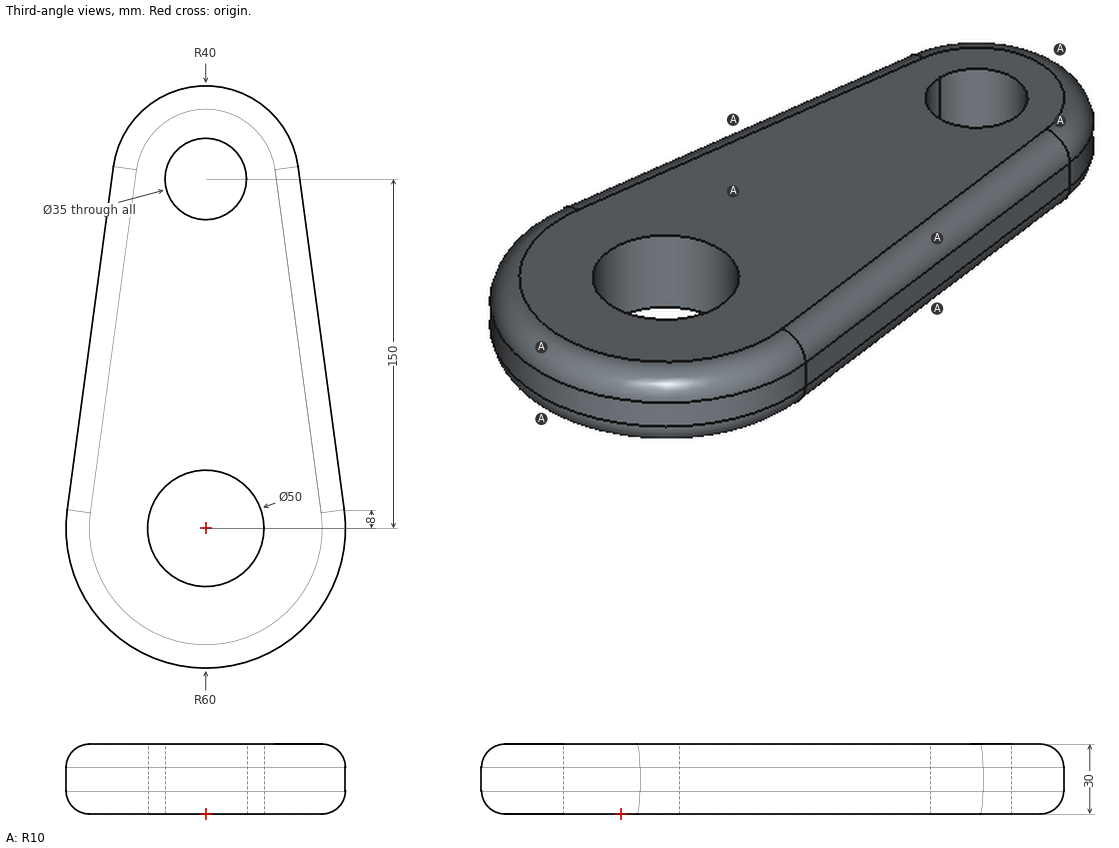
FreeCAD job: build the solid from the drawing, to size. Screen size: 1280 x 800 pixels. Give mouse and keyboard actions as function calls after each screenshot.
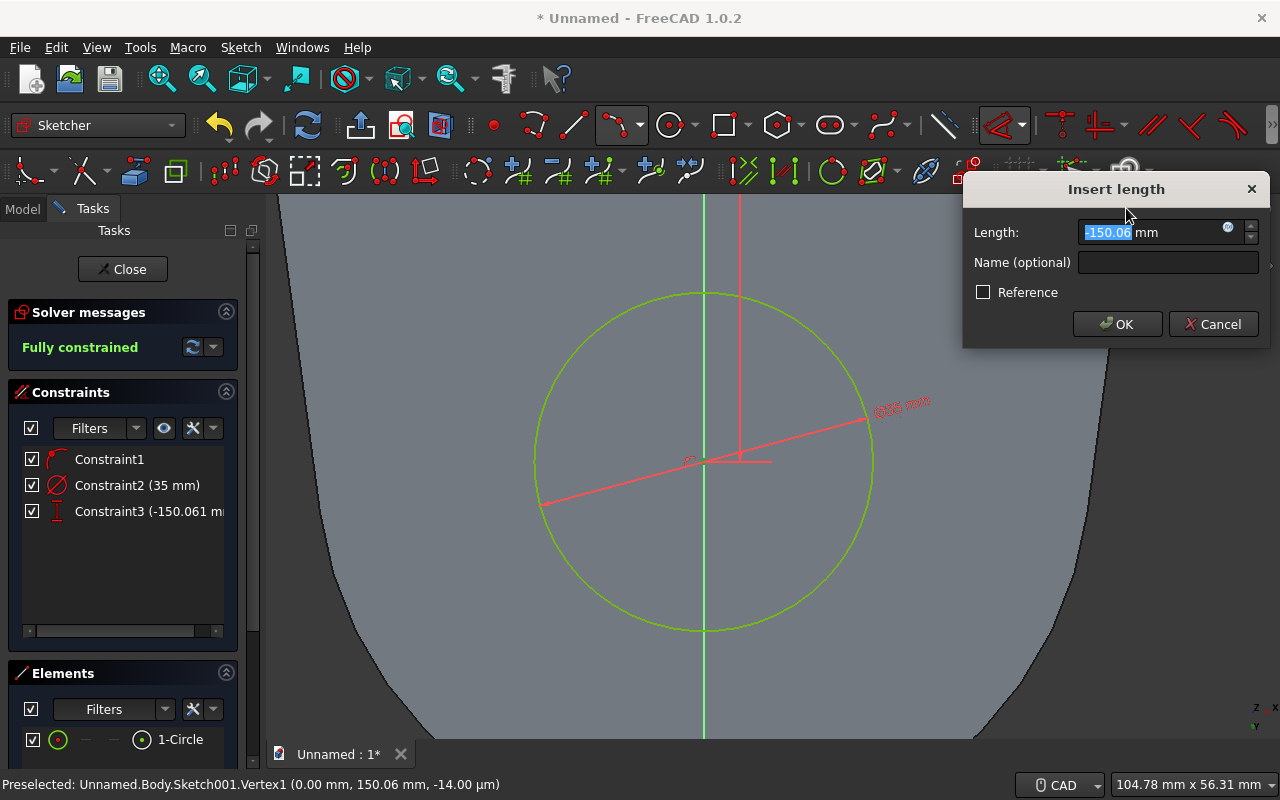
text(-150)
key(Return)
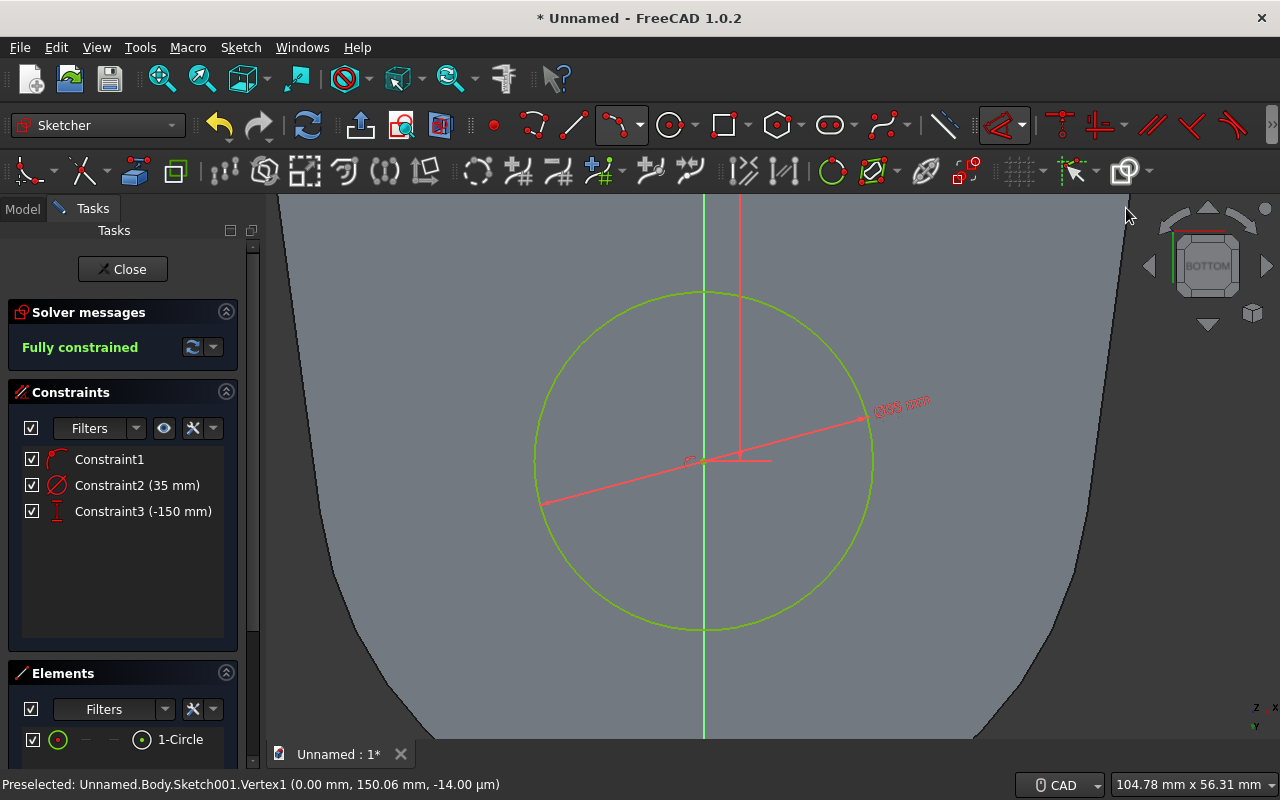
click(123, 269)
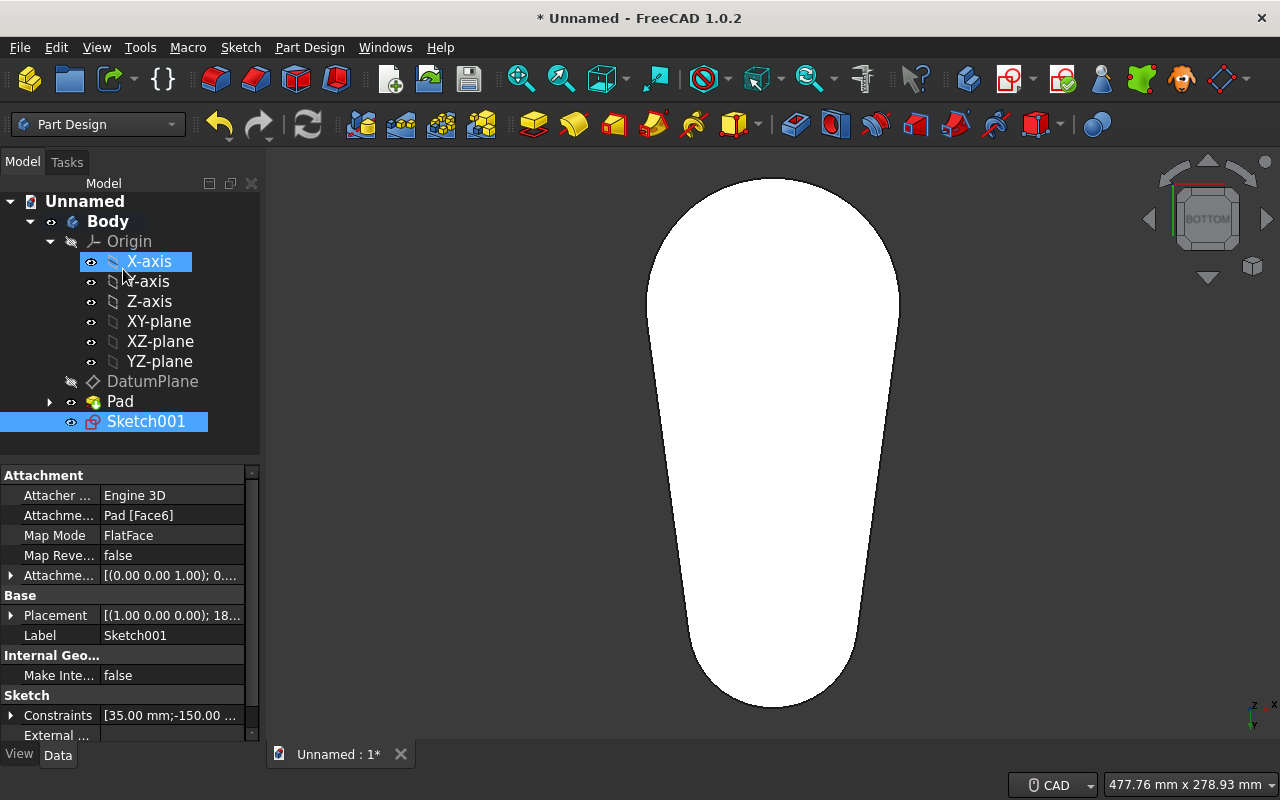
click(836, 124)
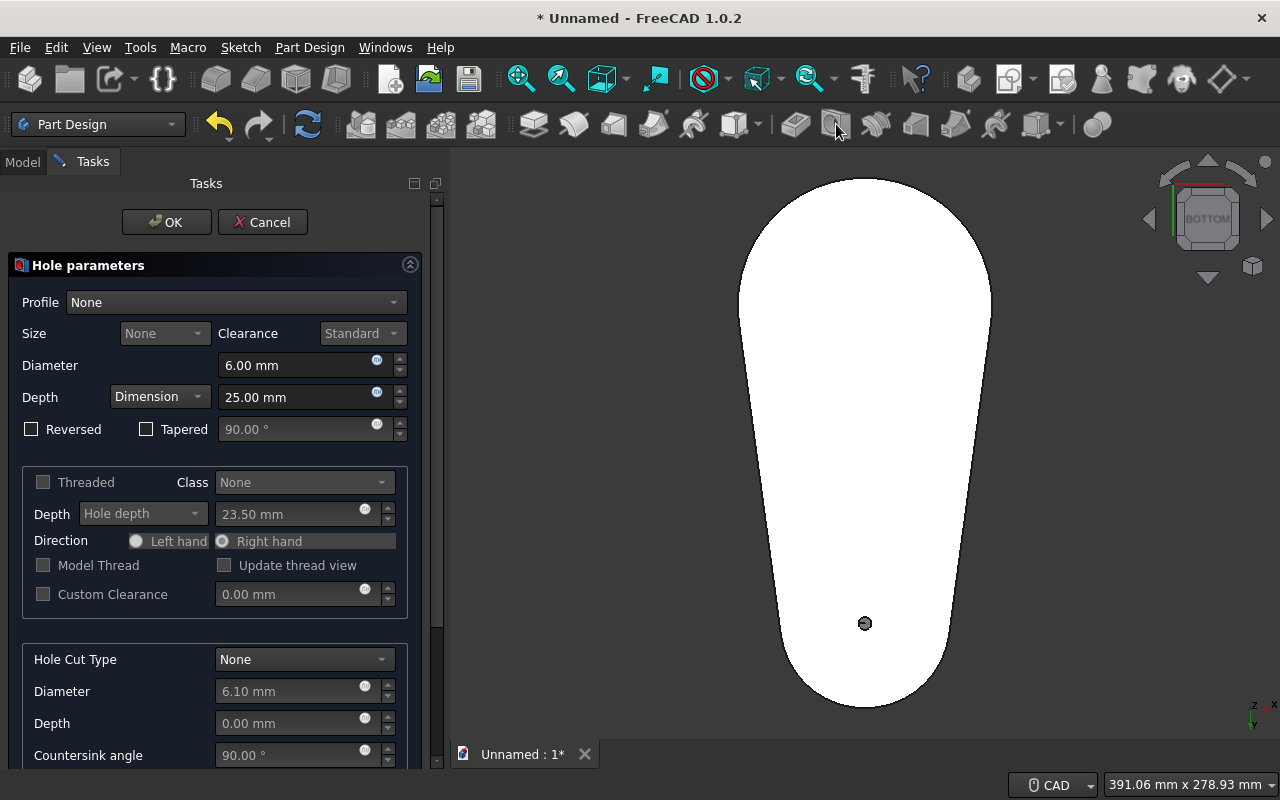
triple_click(305, 365)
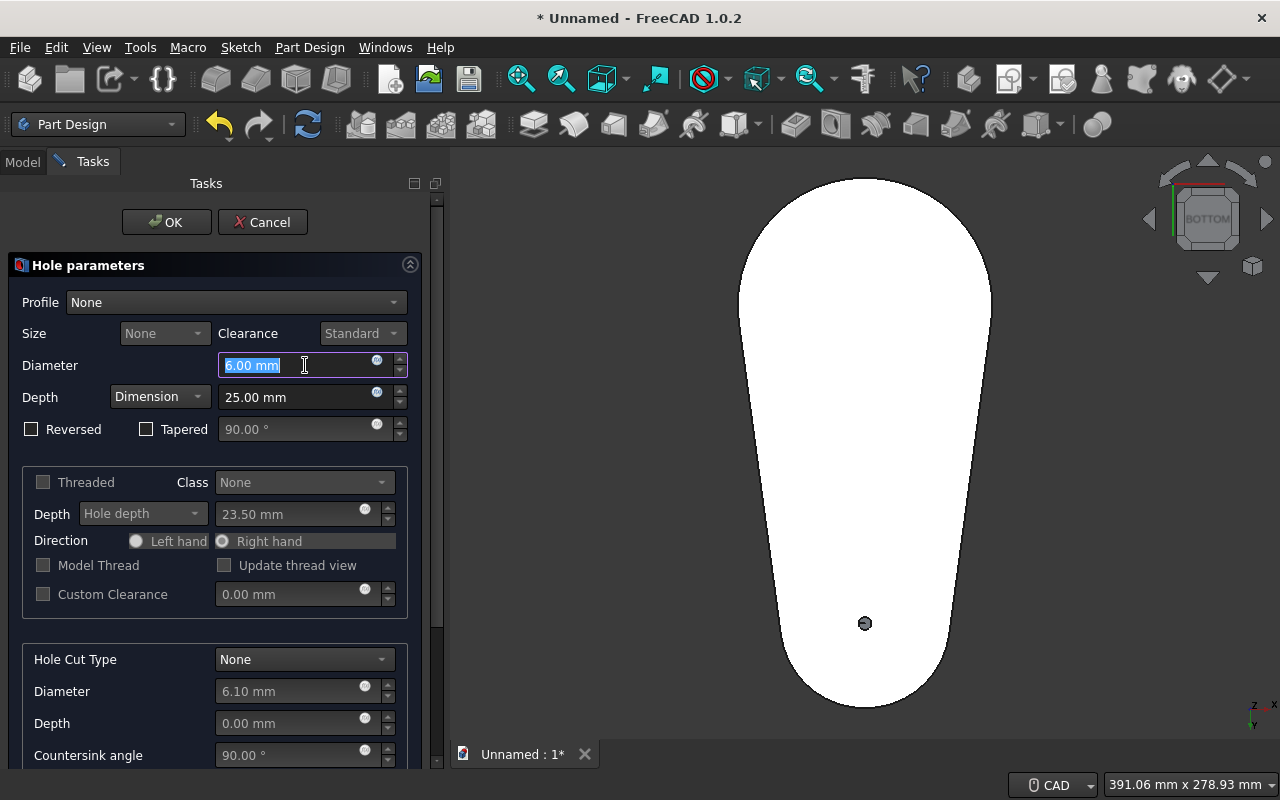
text(35)
key(Tab)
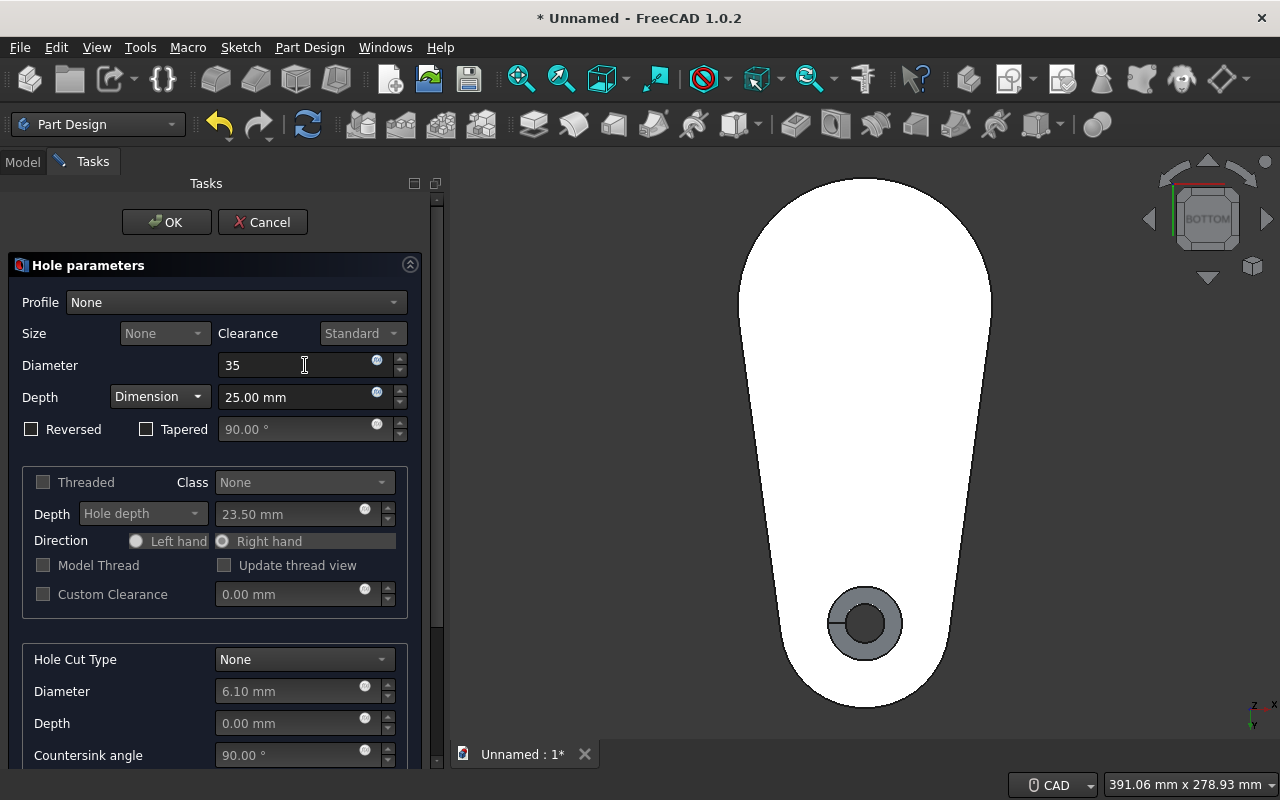
click(161, 396)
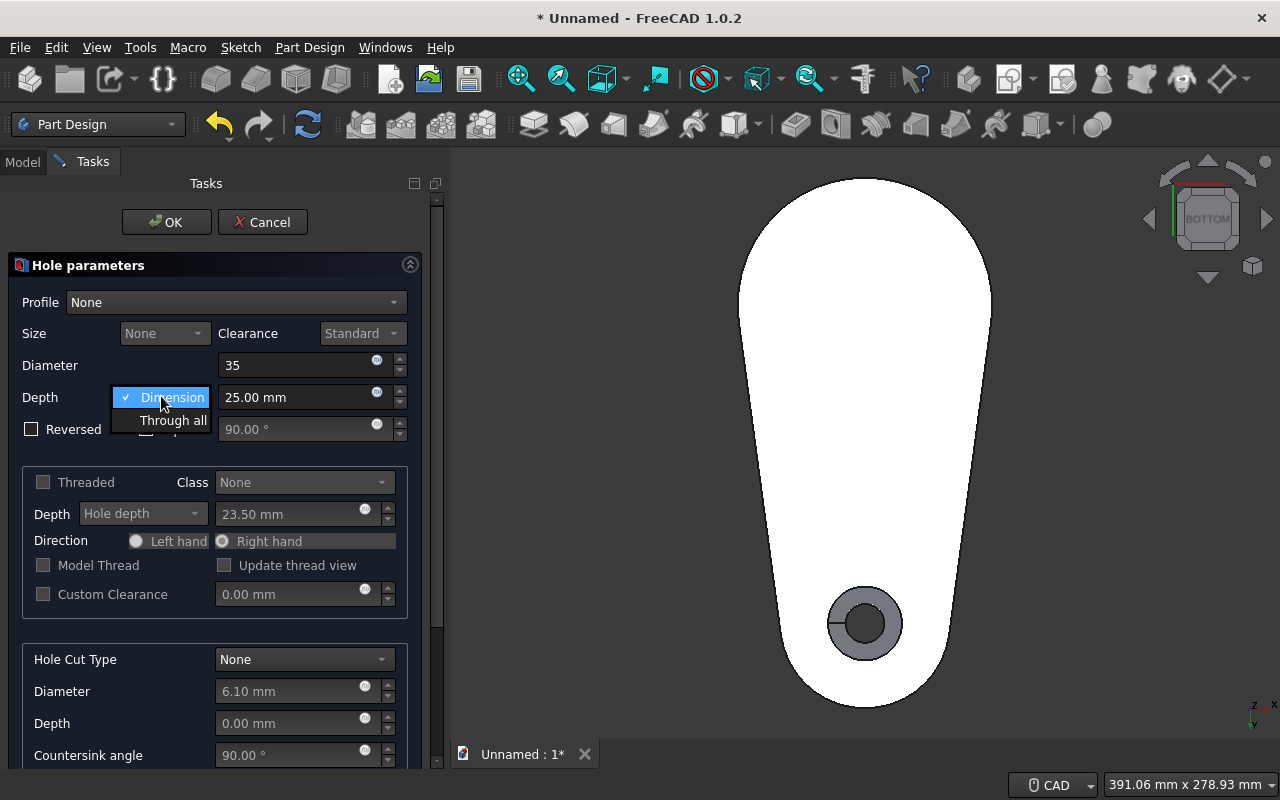
click(160, 420)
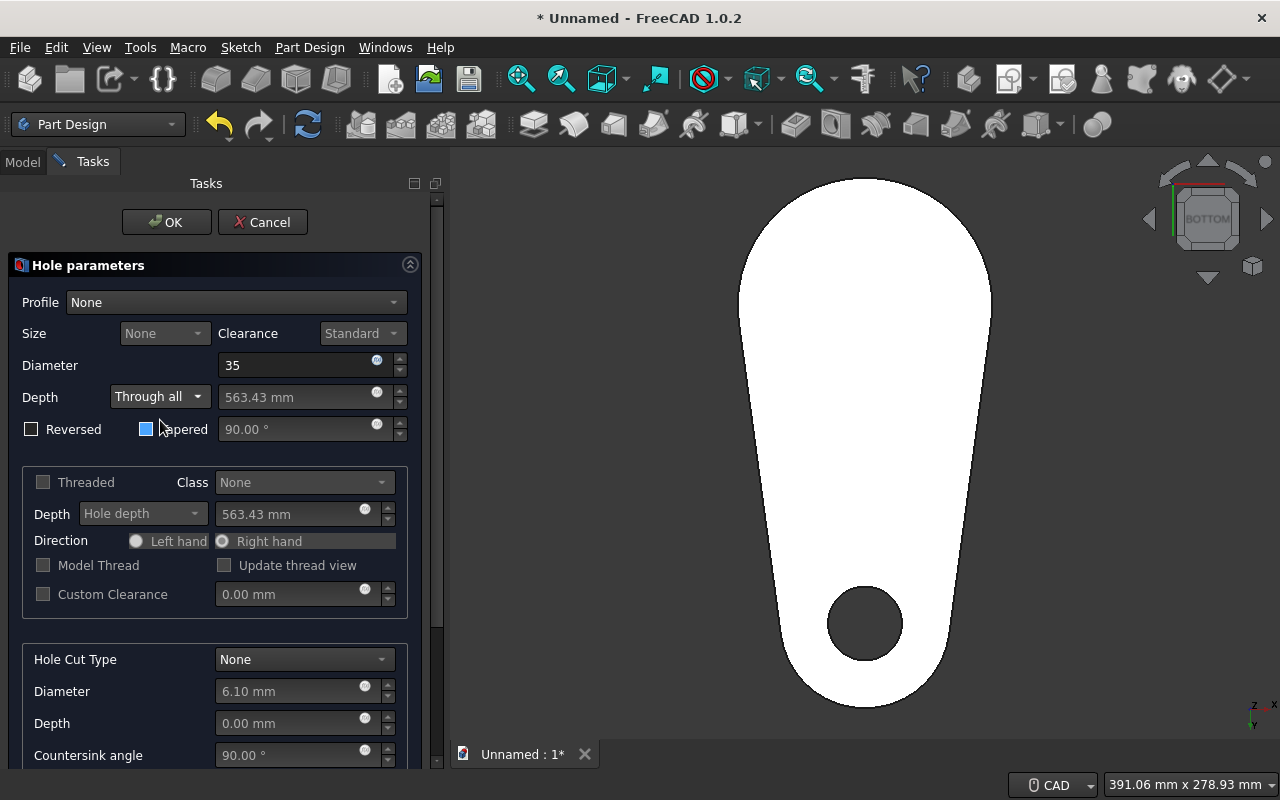
click(167, 222)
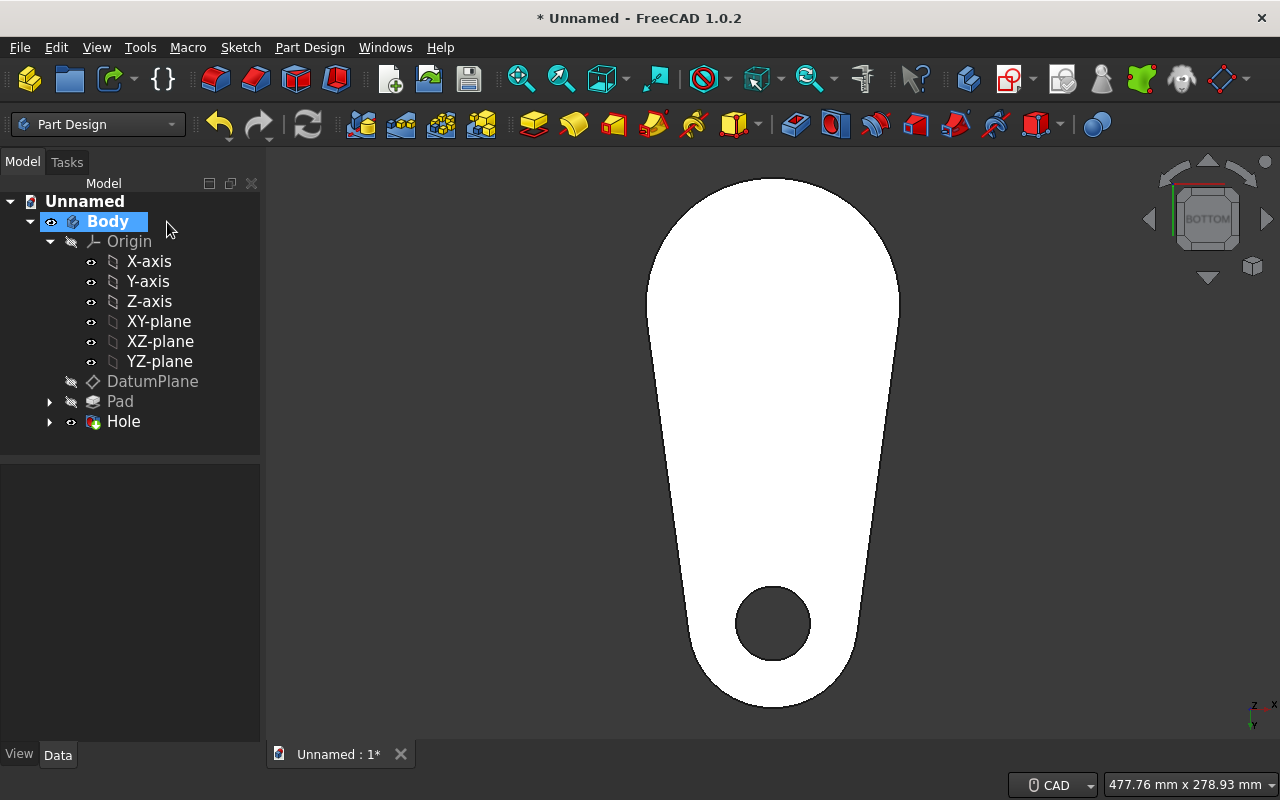
click(1010, 80)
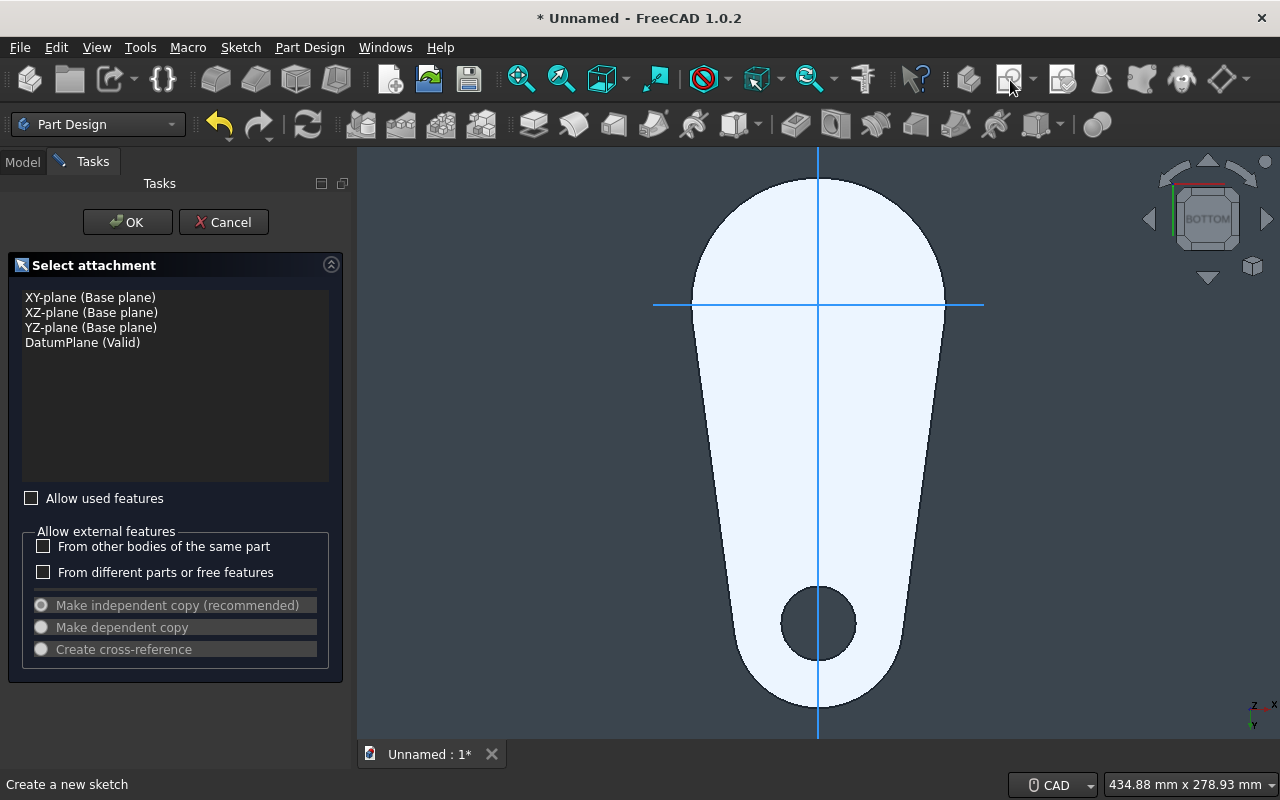
click(82, 298)